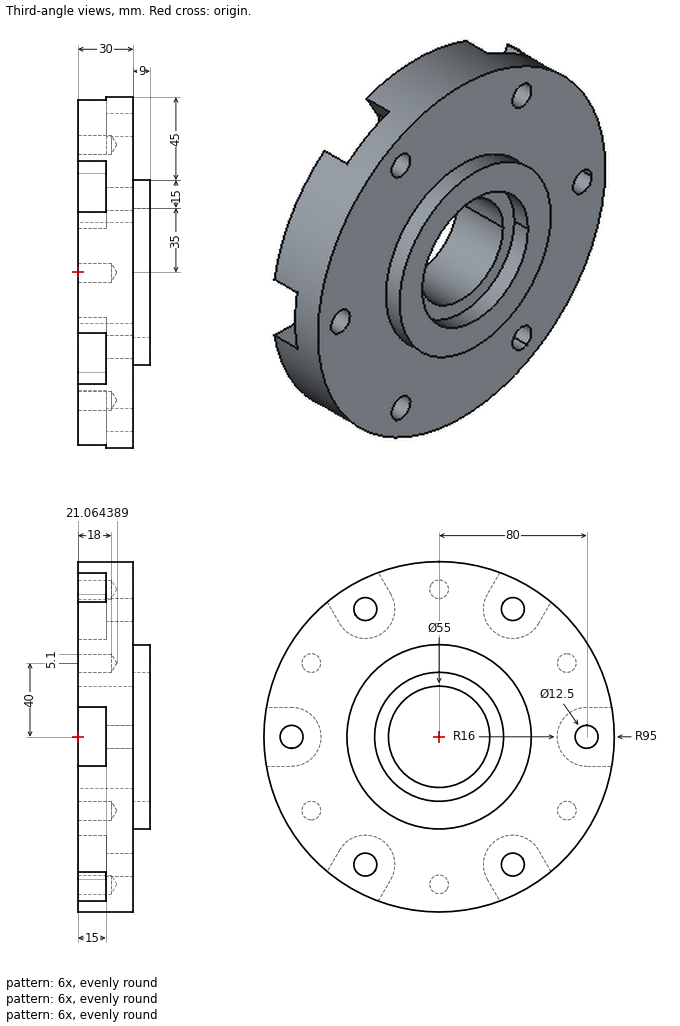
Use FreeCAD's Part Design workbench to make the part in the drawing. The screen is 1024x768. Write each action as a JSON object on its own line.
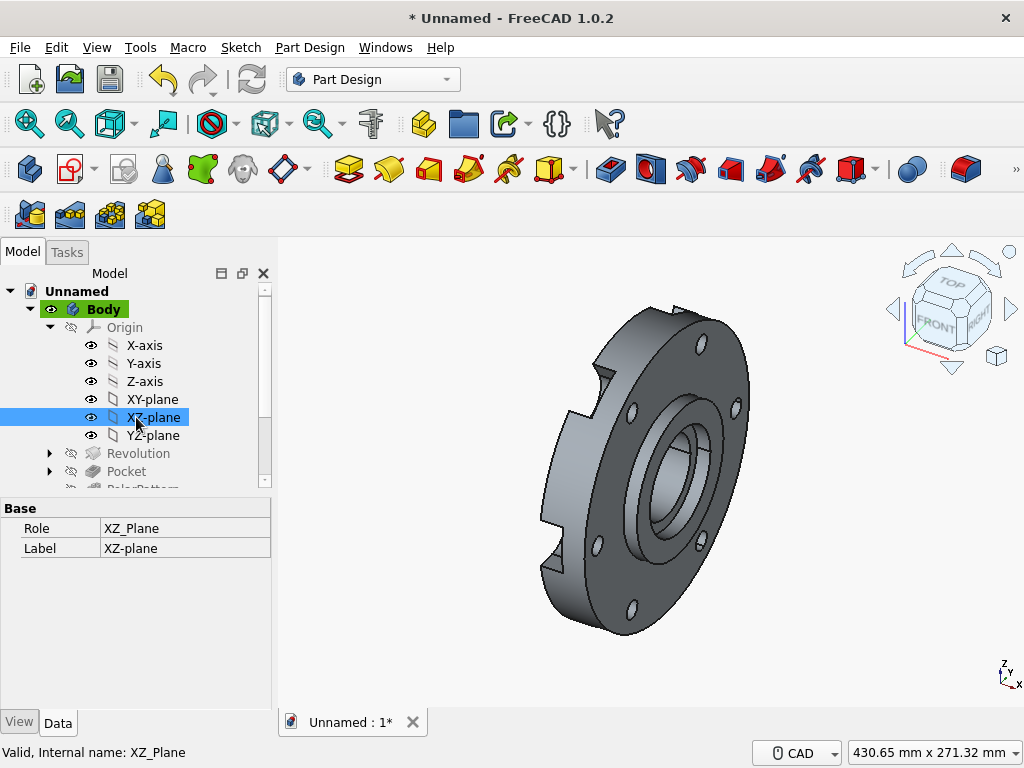
{"action": "left_click", "coordinate": [284, 170]}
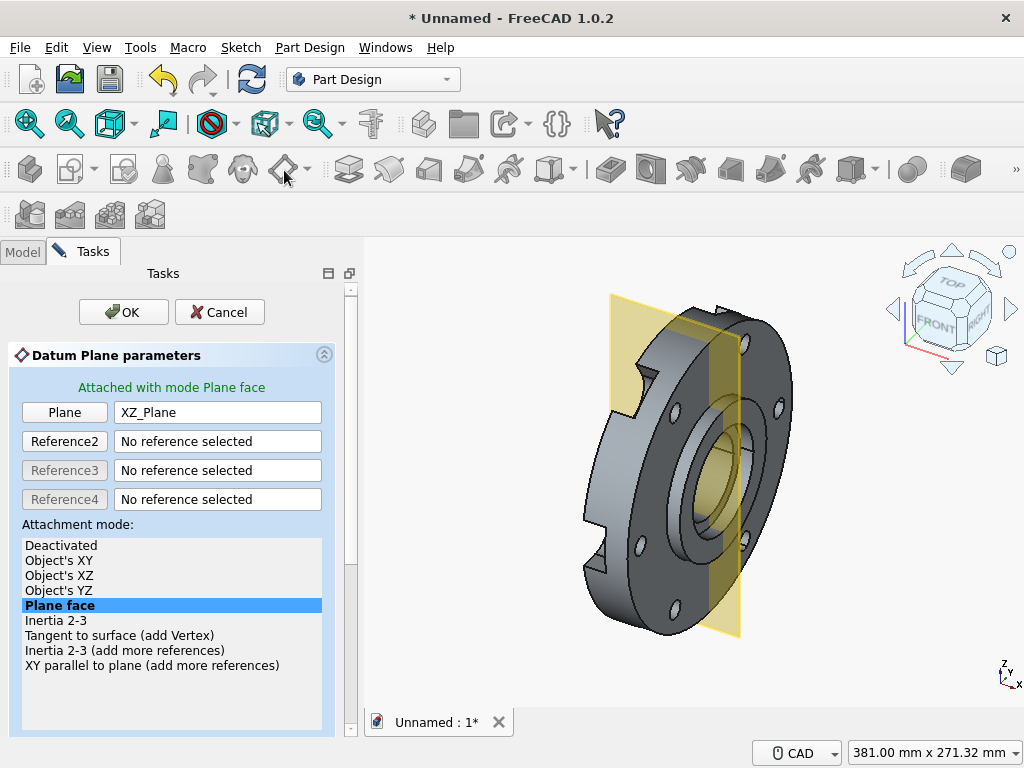
{"action": "scroll", "coordinate": [351, 510], "scroll_direction": "down", "scroll_amount": 3}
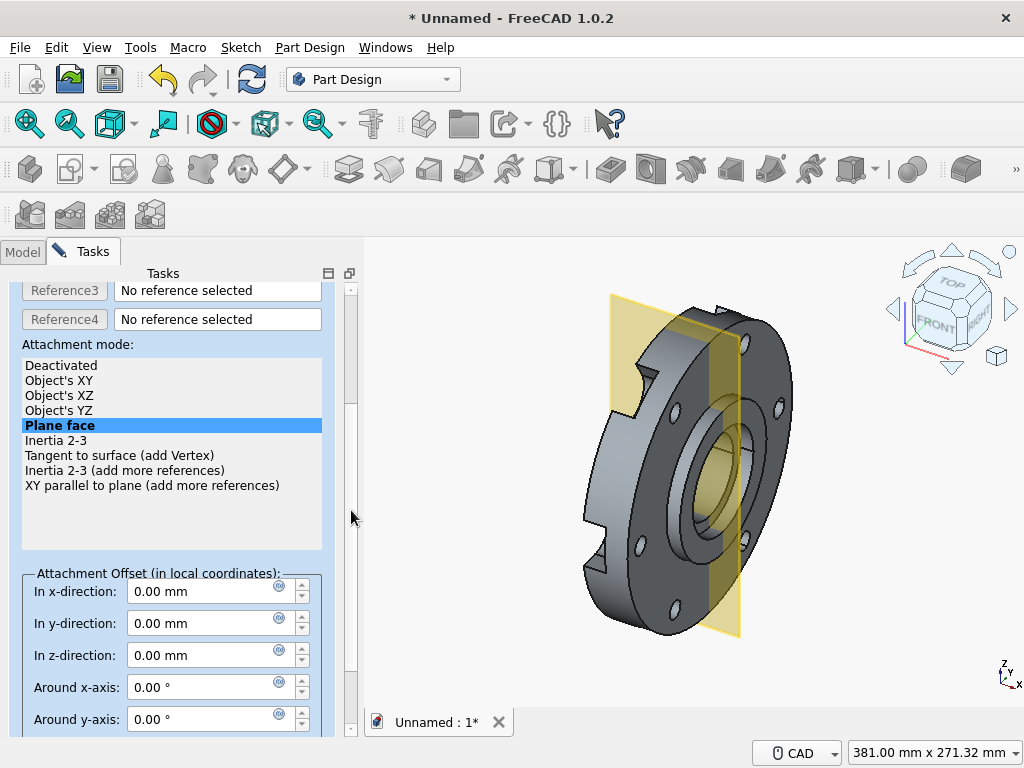
{"action": "triple_click", "coordinate": [210, 655]}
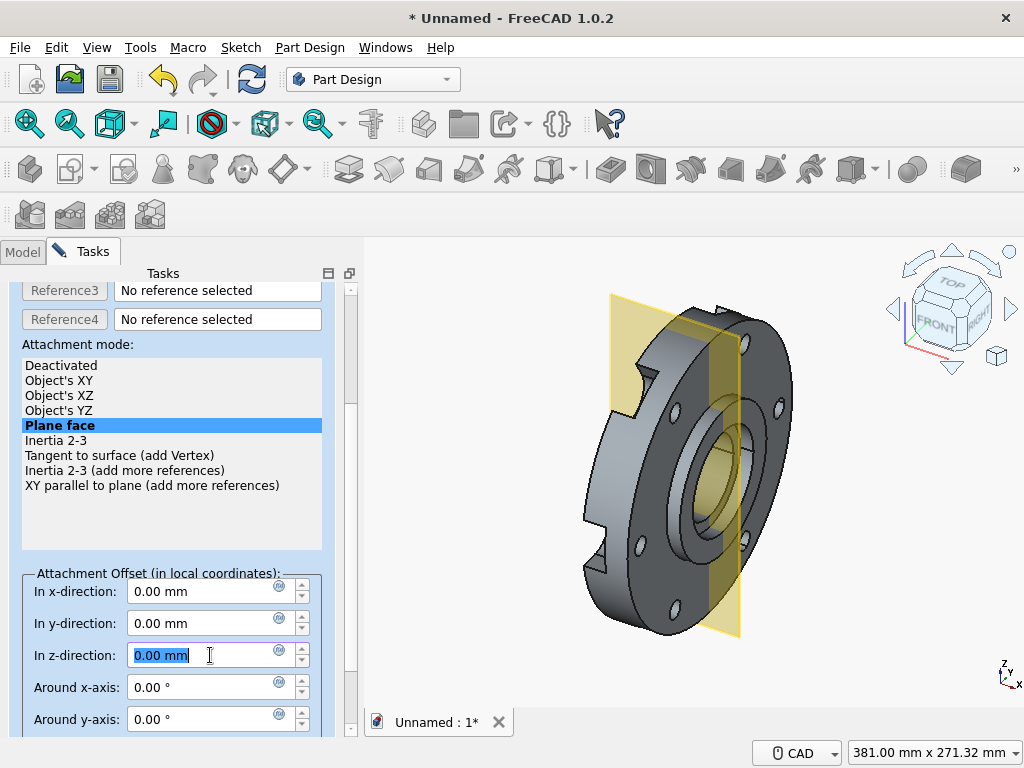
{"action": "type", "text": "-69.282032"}
{"action": "key", "text": "Tab"}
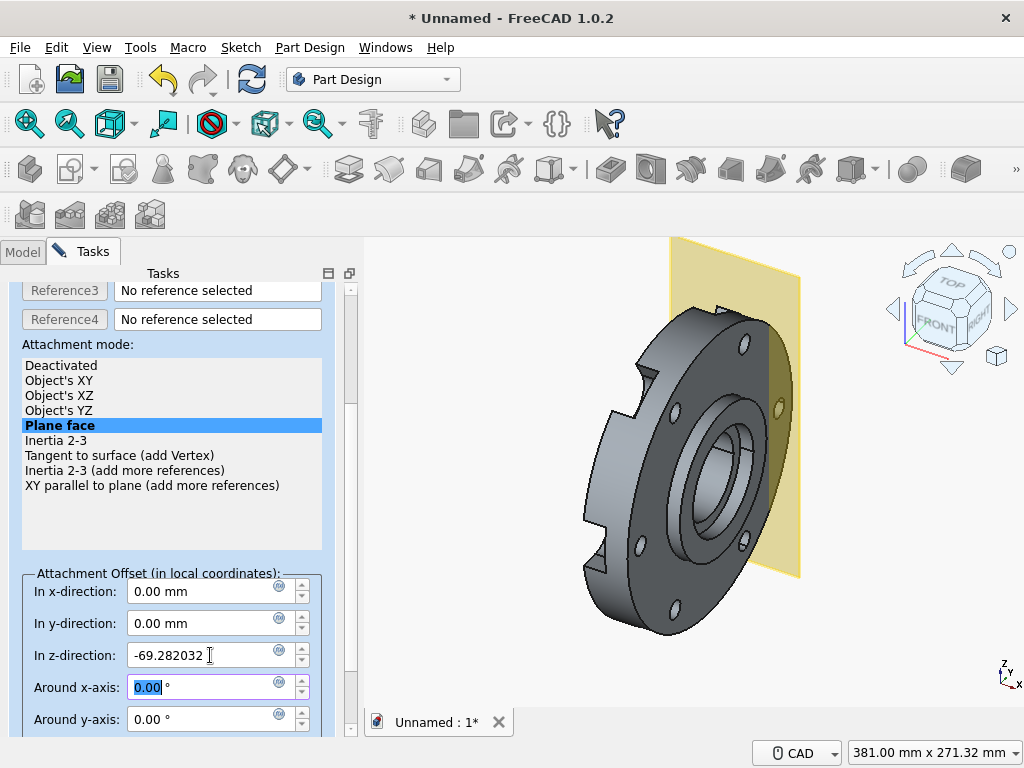
{"action": "scroll", "coordinate": [351, 510], "scroll_direction": "up", "scroll_amount": 4}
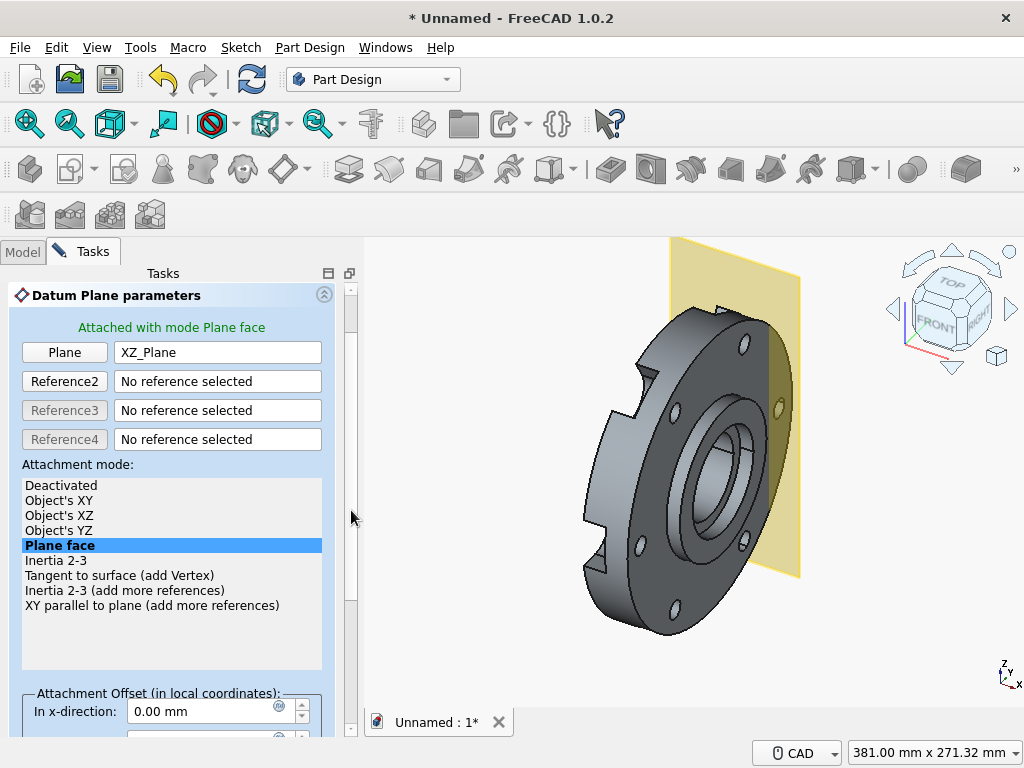
{"action": "left_click", "coordinate": [124, 312]}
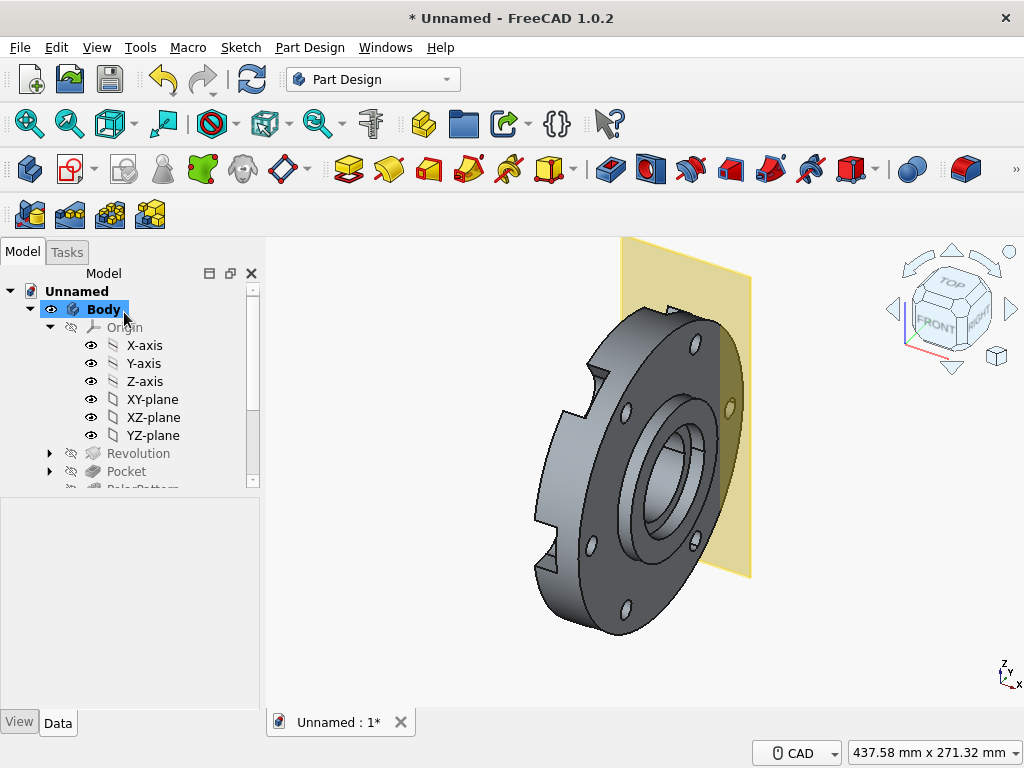
{"action": "scroll", "coordinate": [100, 377], "scroll_direction": "down", "scroll_amount": 3}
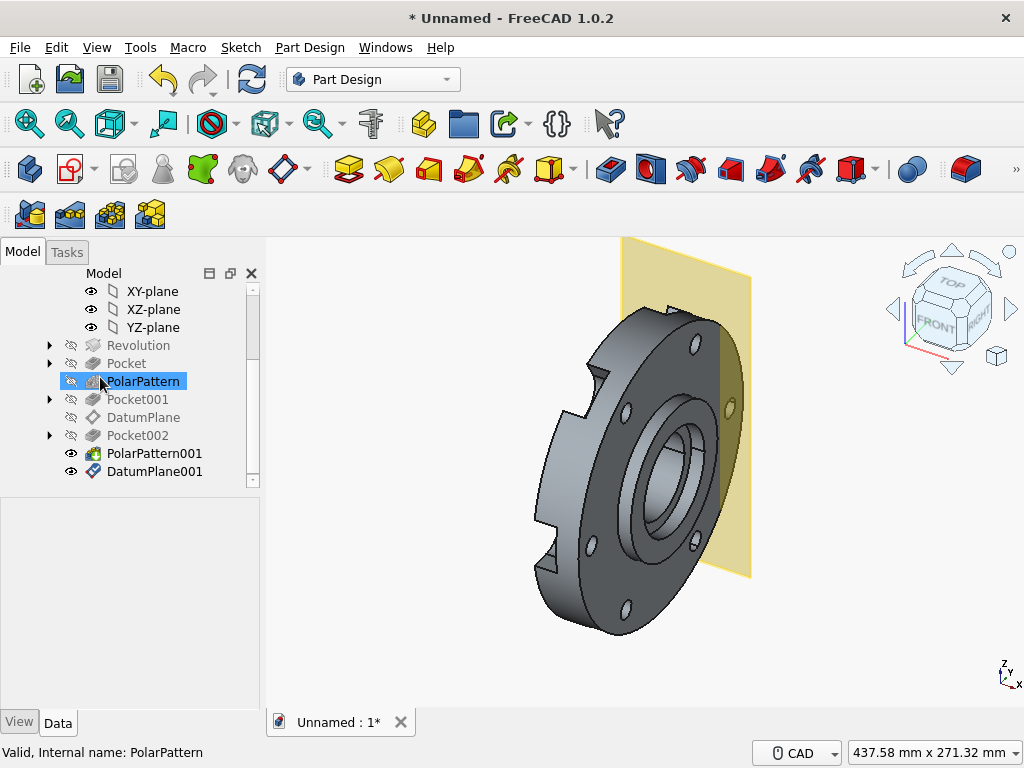
{"action": "left_click", "coordinate": [116, 471]}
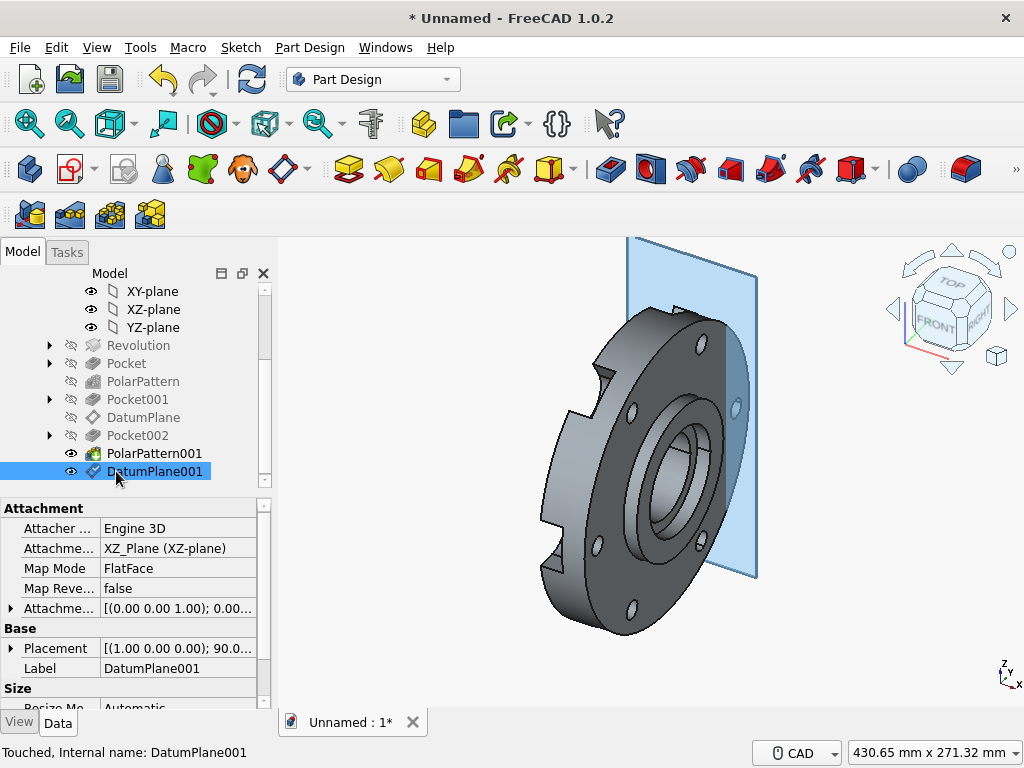
{"action": "left_click", "coordinate": [70, 170]}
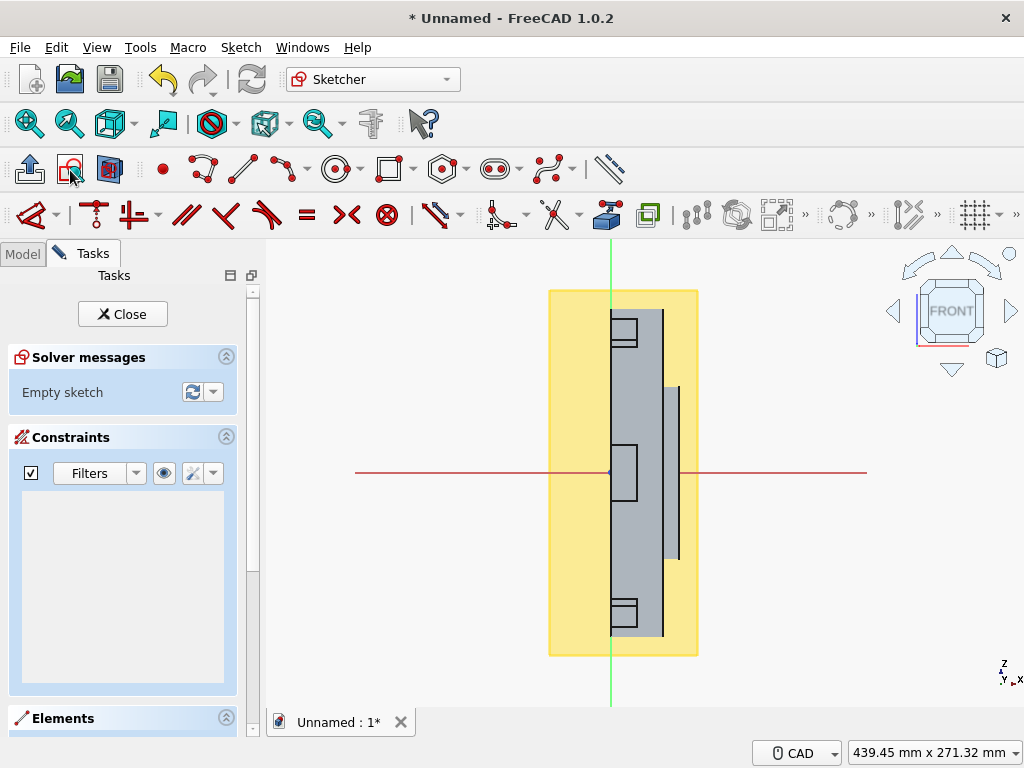
{"action": "left_click", "coordinate": [110, 170]}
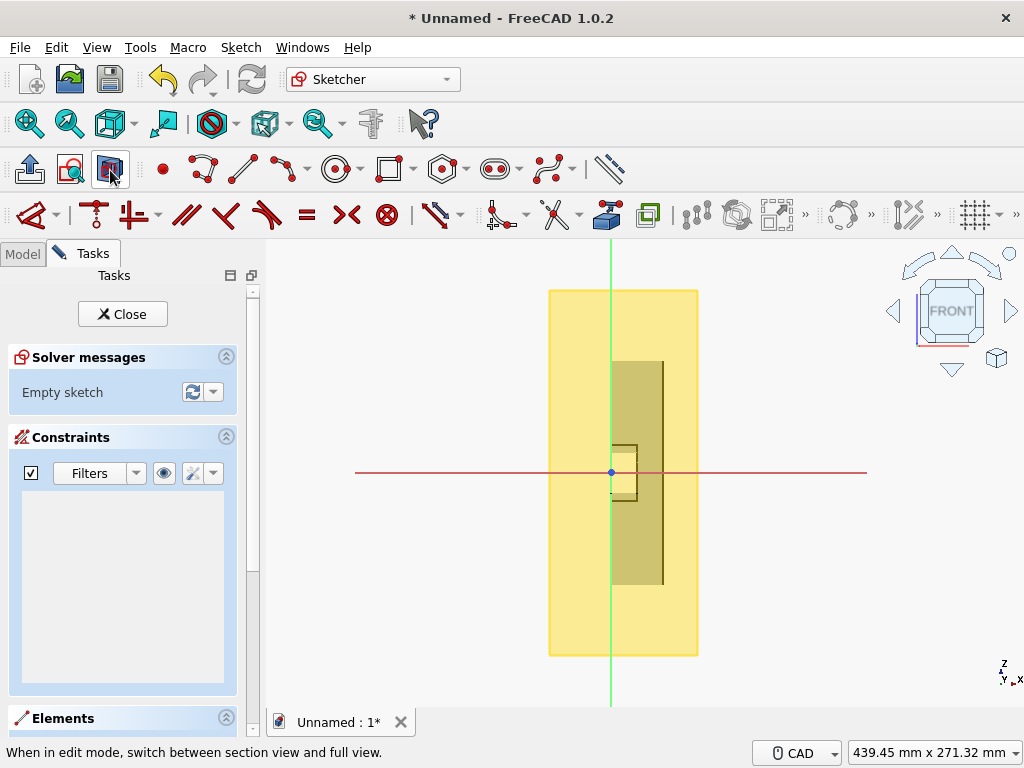
{"action": "scroll", "coordinate": [657, 421], "scroll_direction": "up", "scroll_amount": 7}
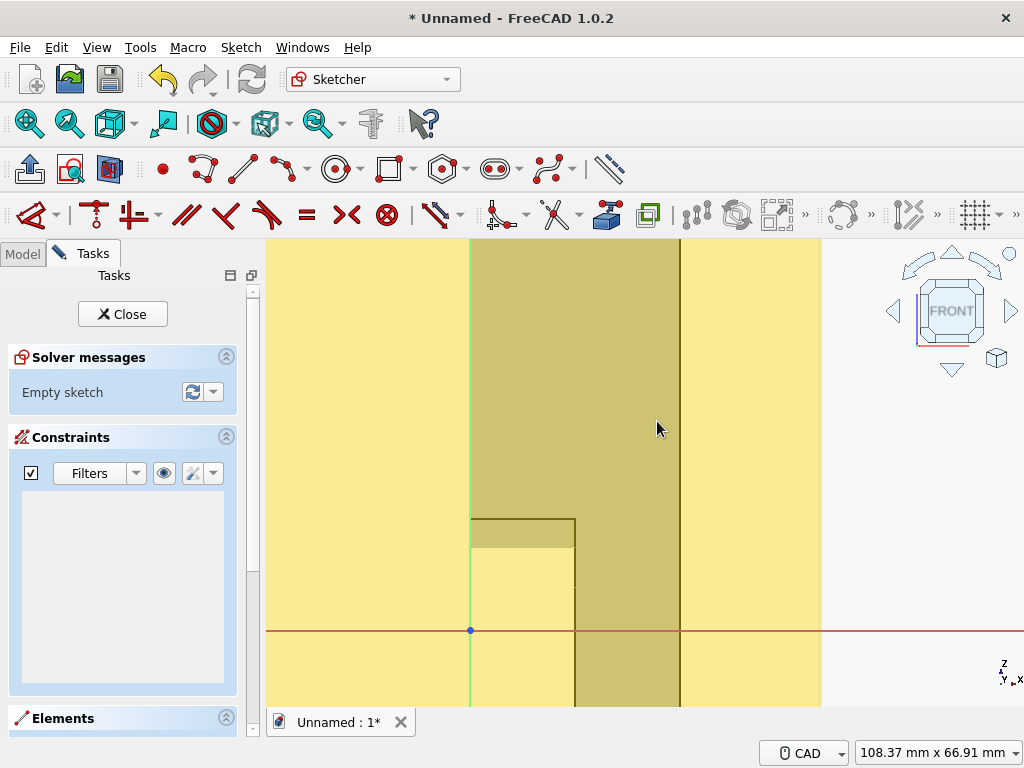
{"action": "left_click", "coordinate": [204, 170]}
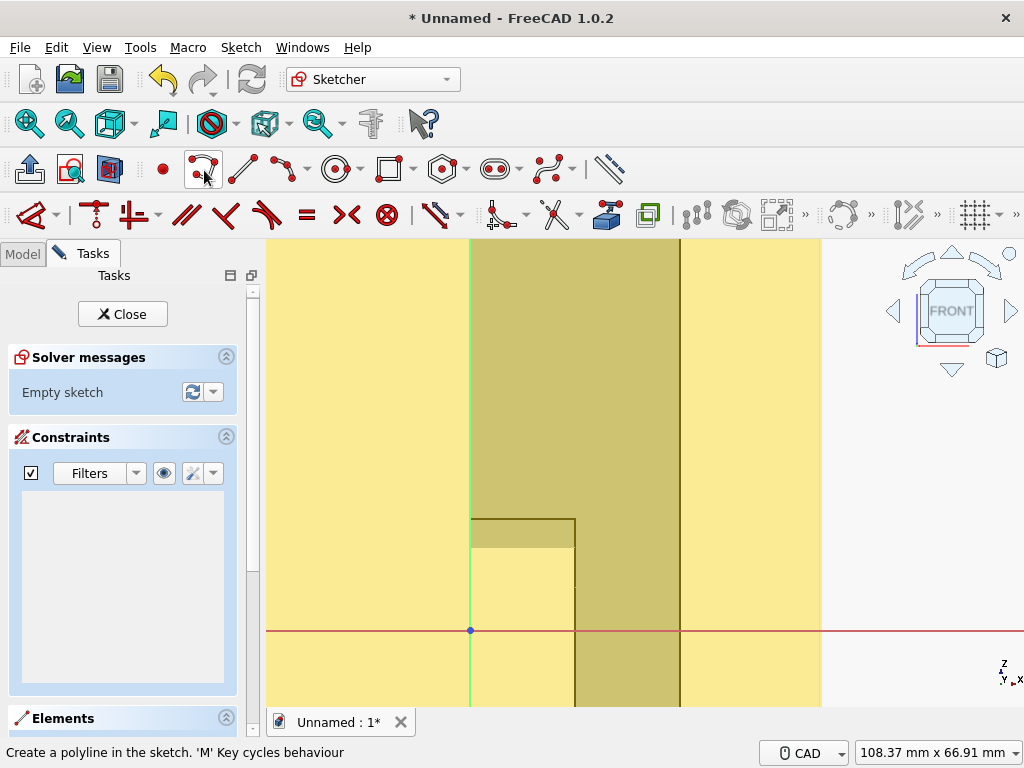
{"action": "left_click", "coordinate": [470, 351]}
{"action": "left_click", "coordinate": [479, 315]}
{"action": "left_click", "coordinate": [596, 315]}
{"action": "left_click", "coordinate": [618, 351]}
{"action": "left_click", "coordinate": [470, 352]}